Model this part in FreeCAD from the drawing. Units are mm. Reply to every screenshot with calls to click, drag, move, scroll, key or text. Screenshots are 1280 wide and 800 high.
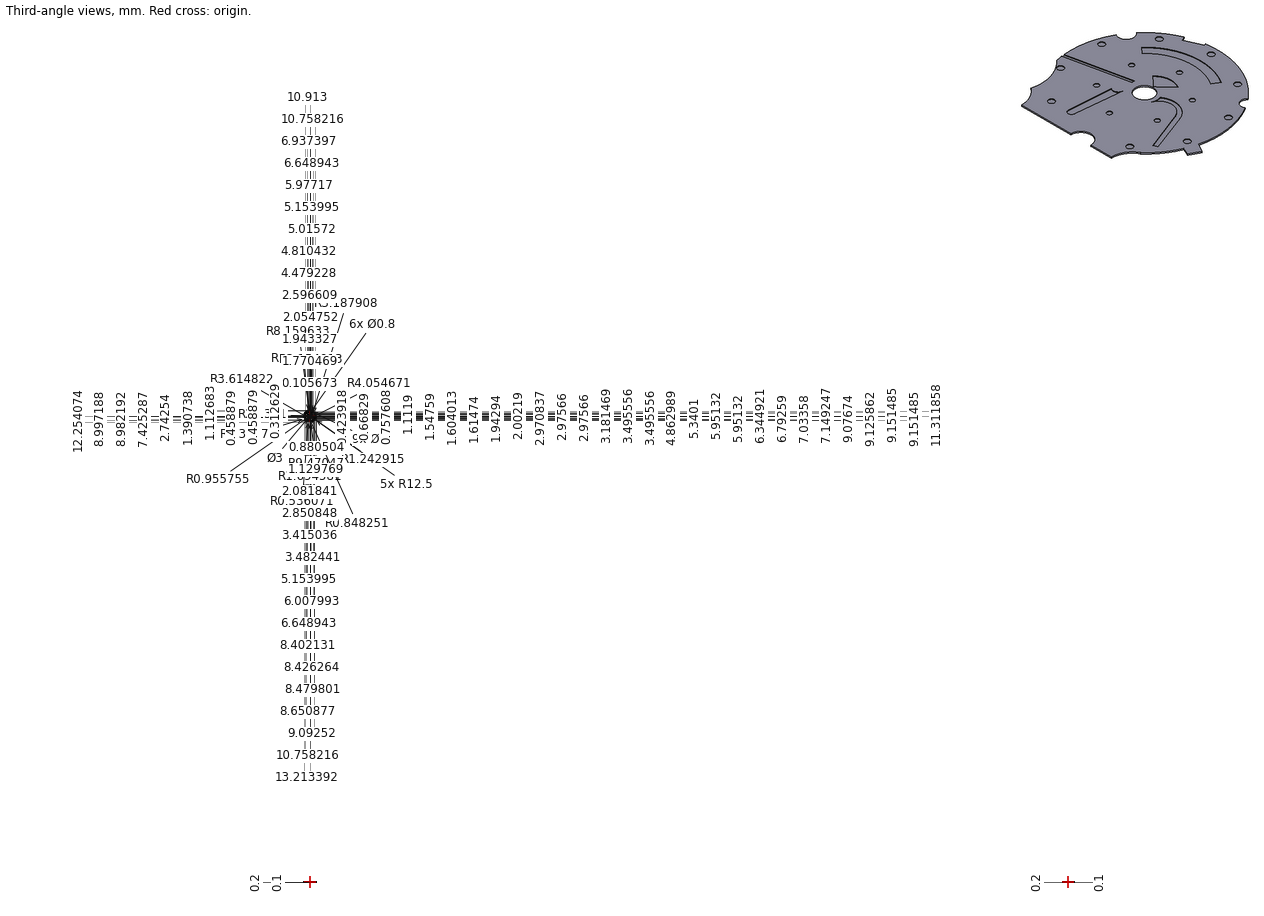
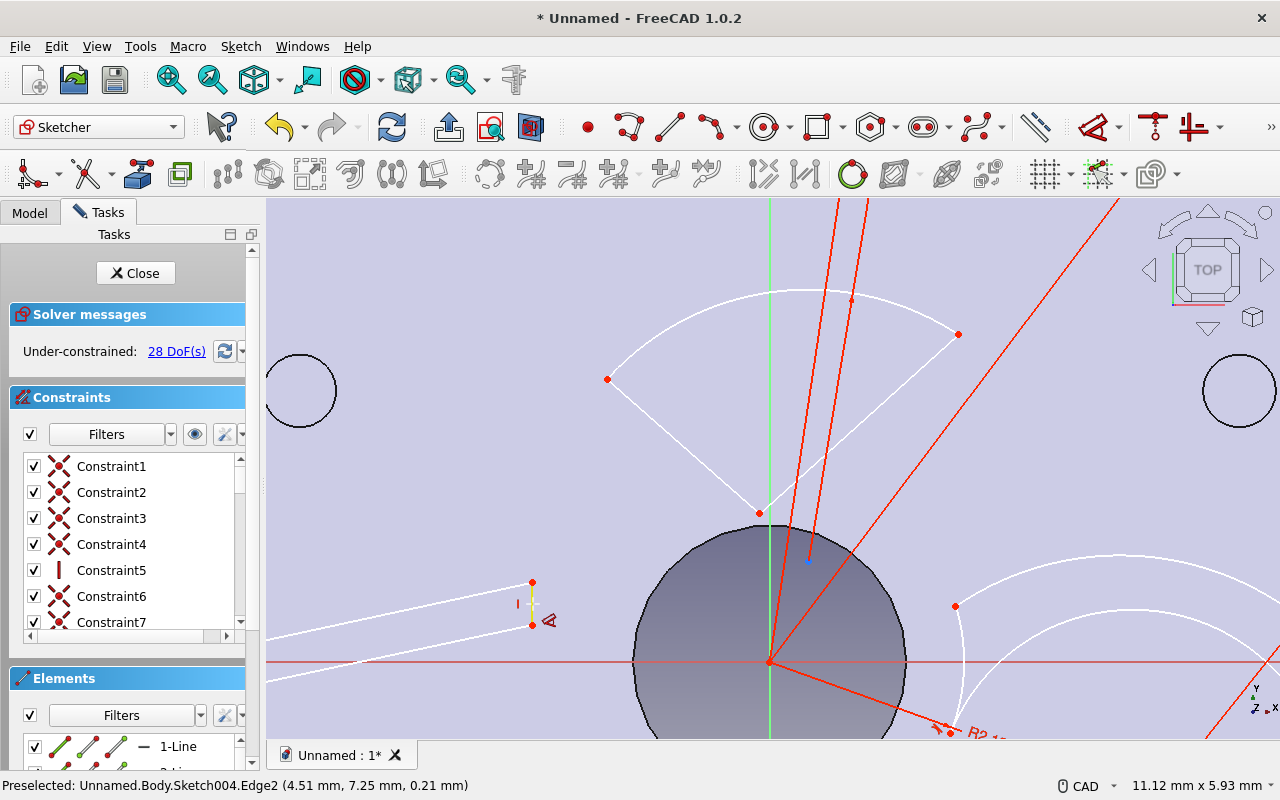
click(532, 604)
click(498, 604)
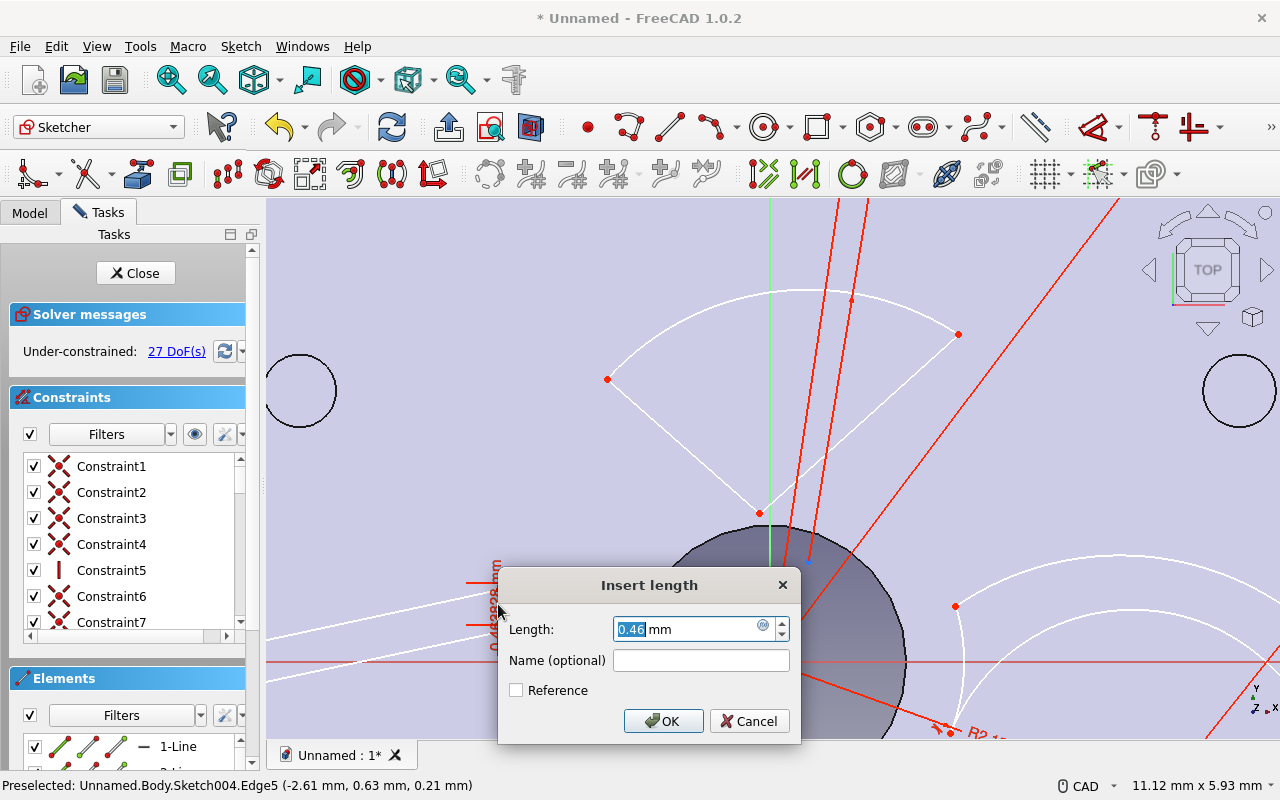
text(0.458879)
key(Return)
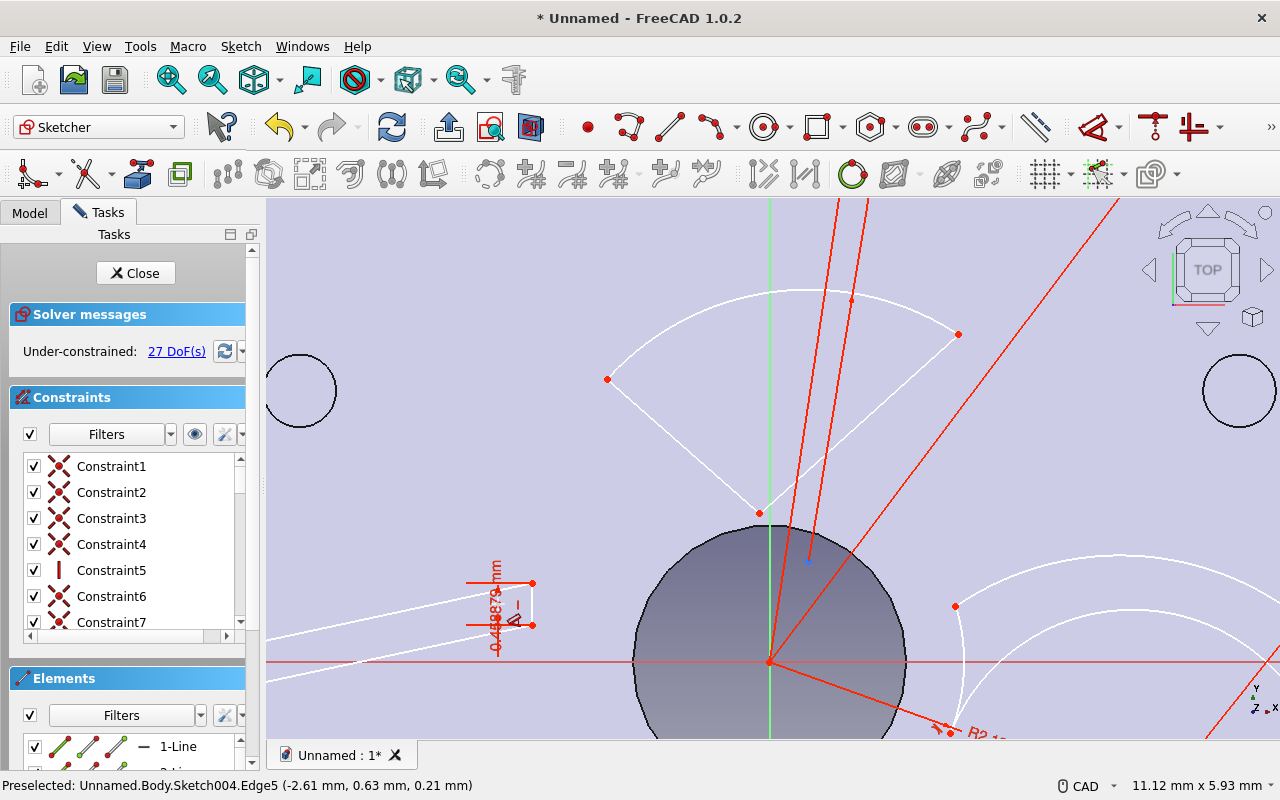
scroll(736, 417, down, 8)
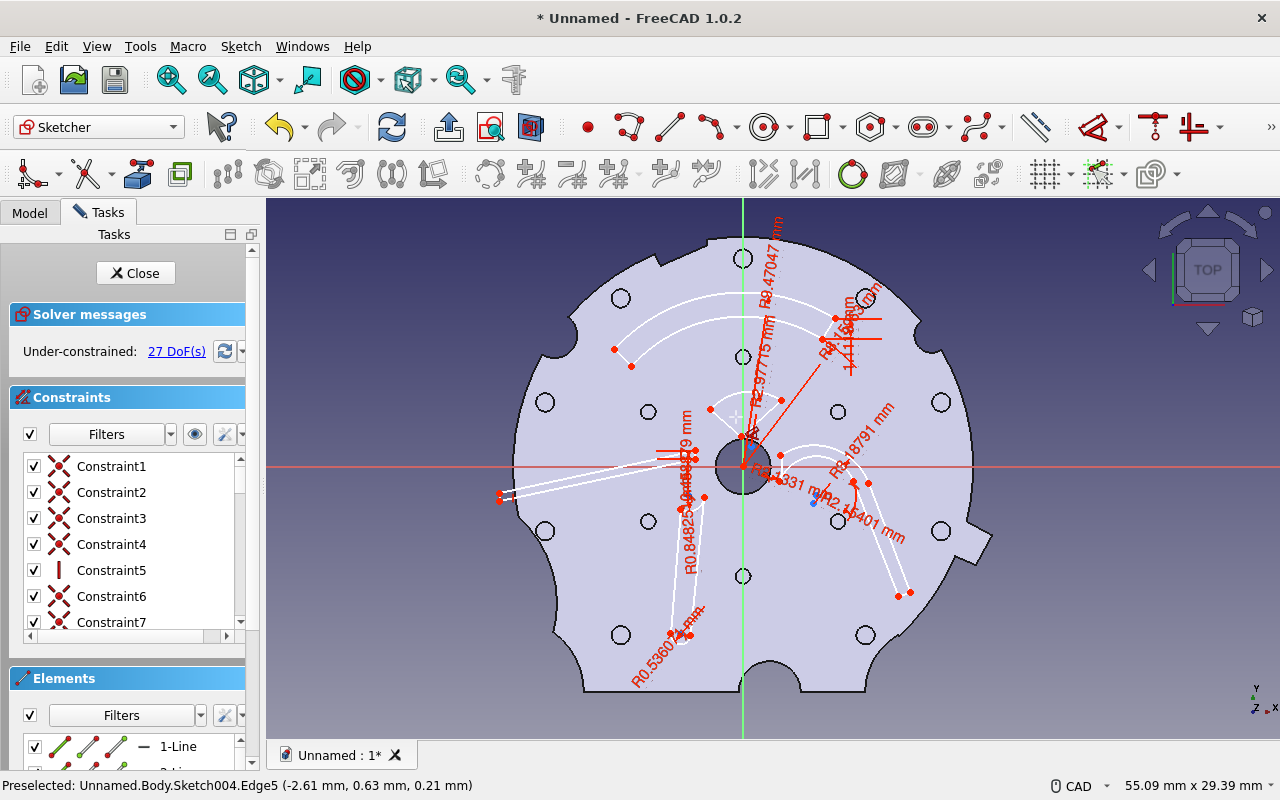
scroll(500, 495, up, 9)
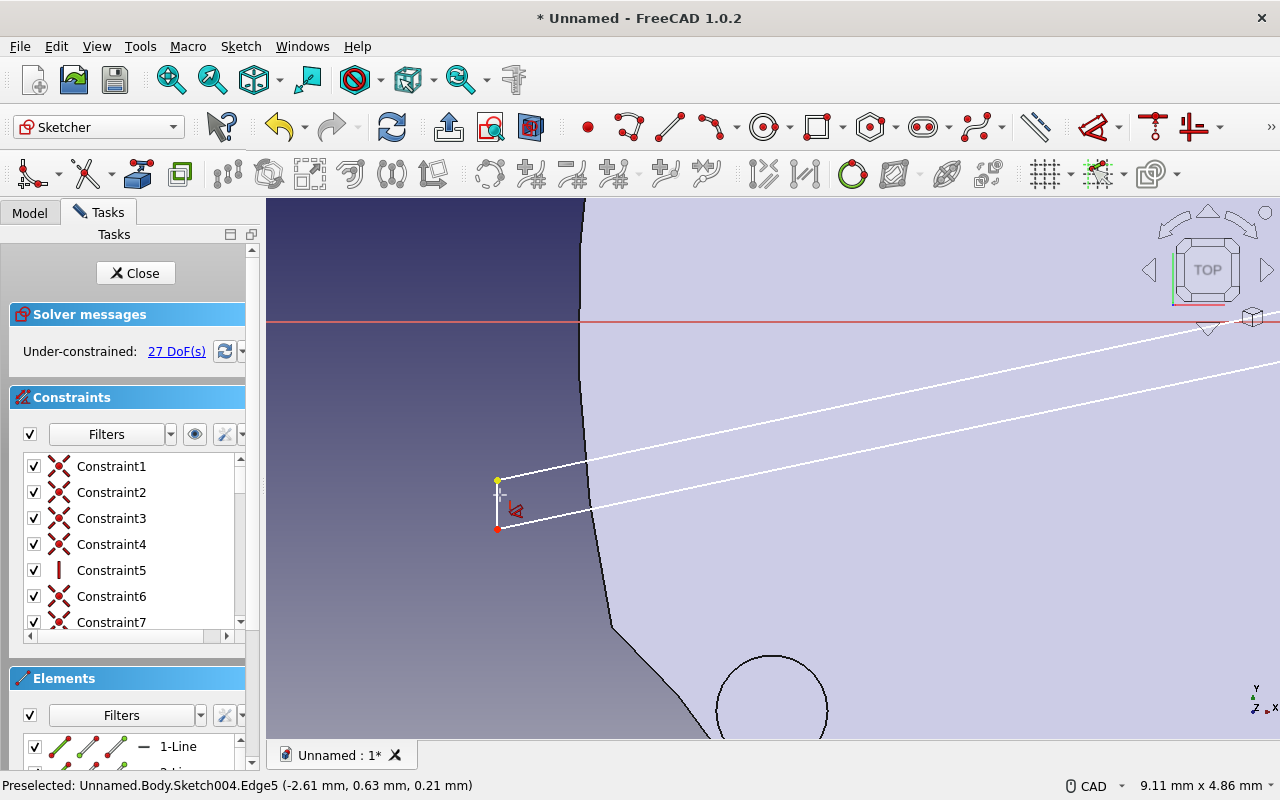
click(497, 495)
click(463, 505)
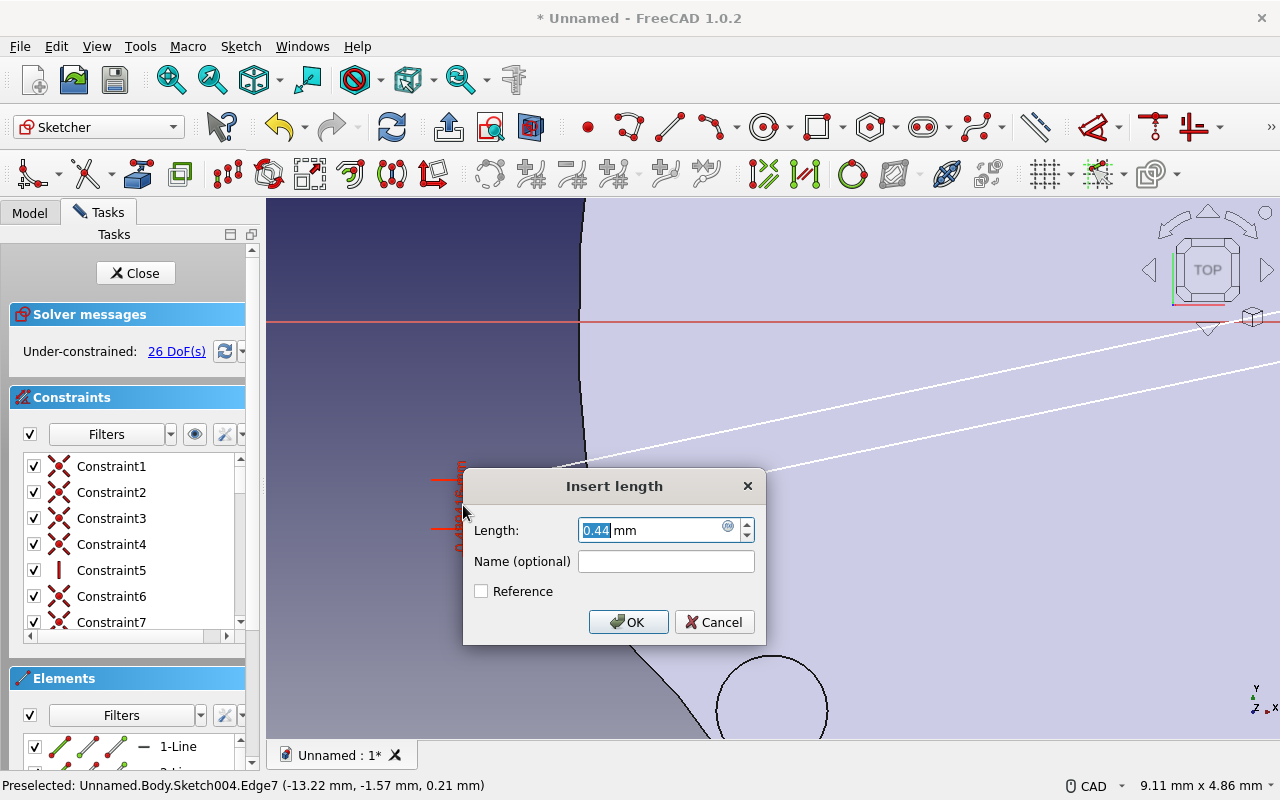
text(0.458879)
key(Return)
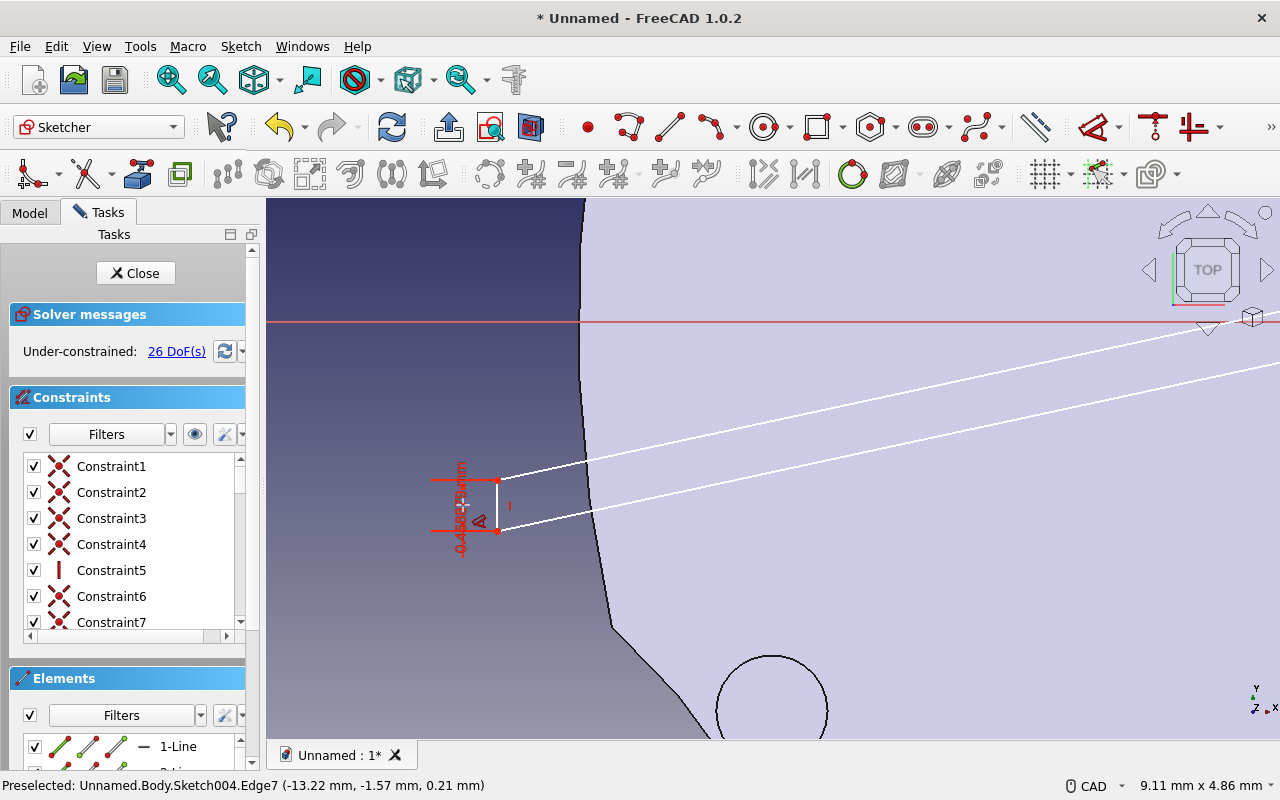
scroll(499, 496, down, 9)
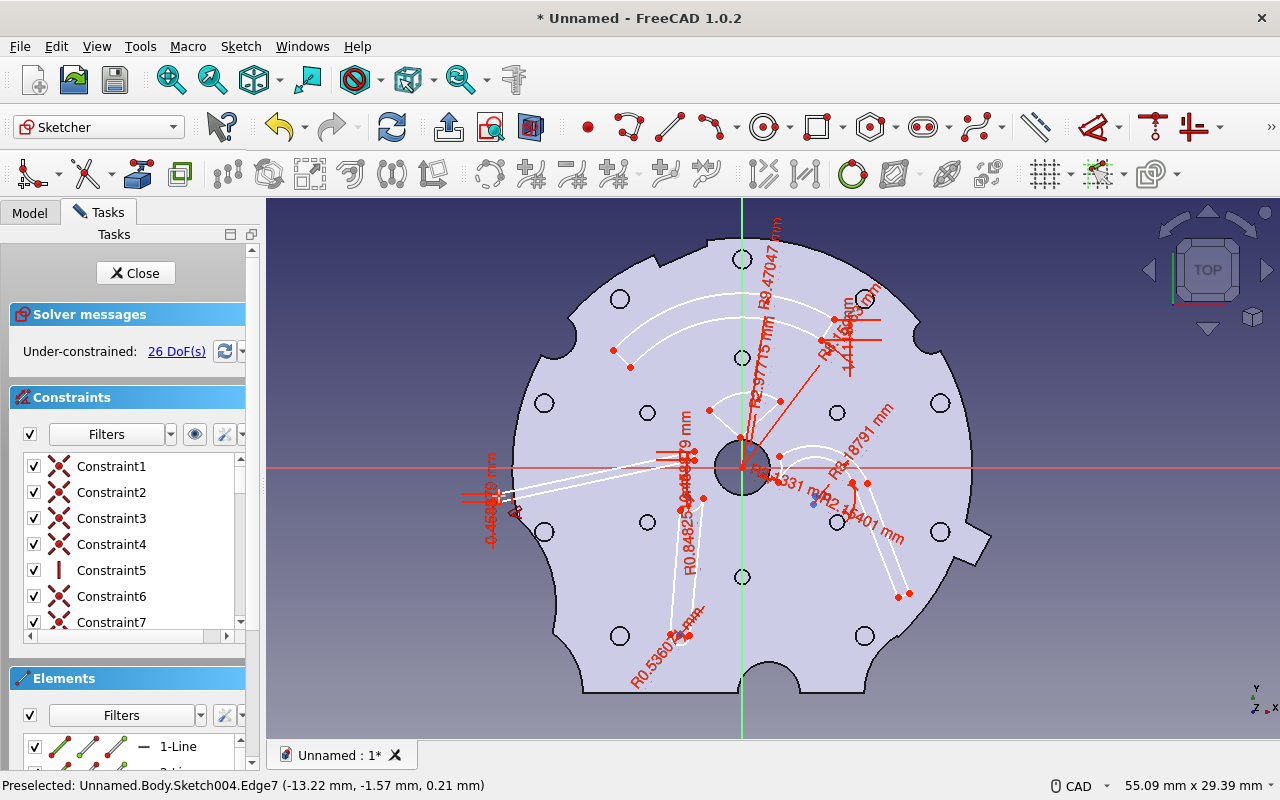
click(631, 367)
click(726, 333)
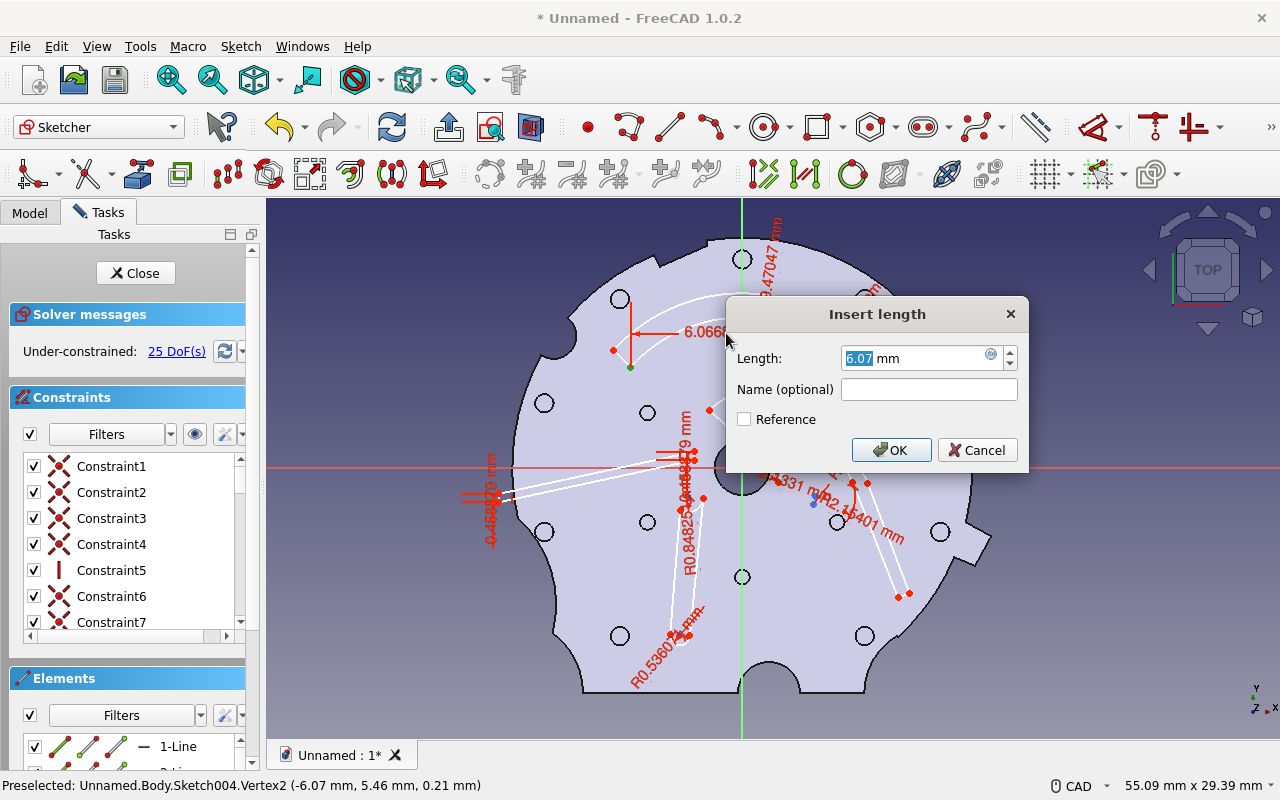
text(5.97717)
key(Return)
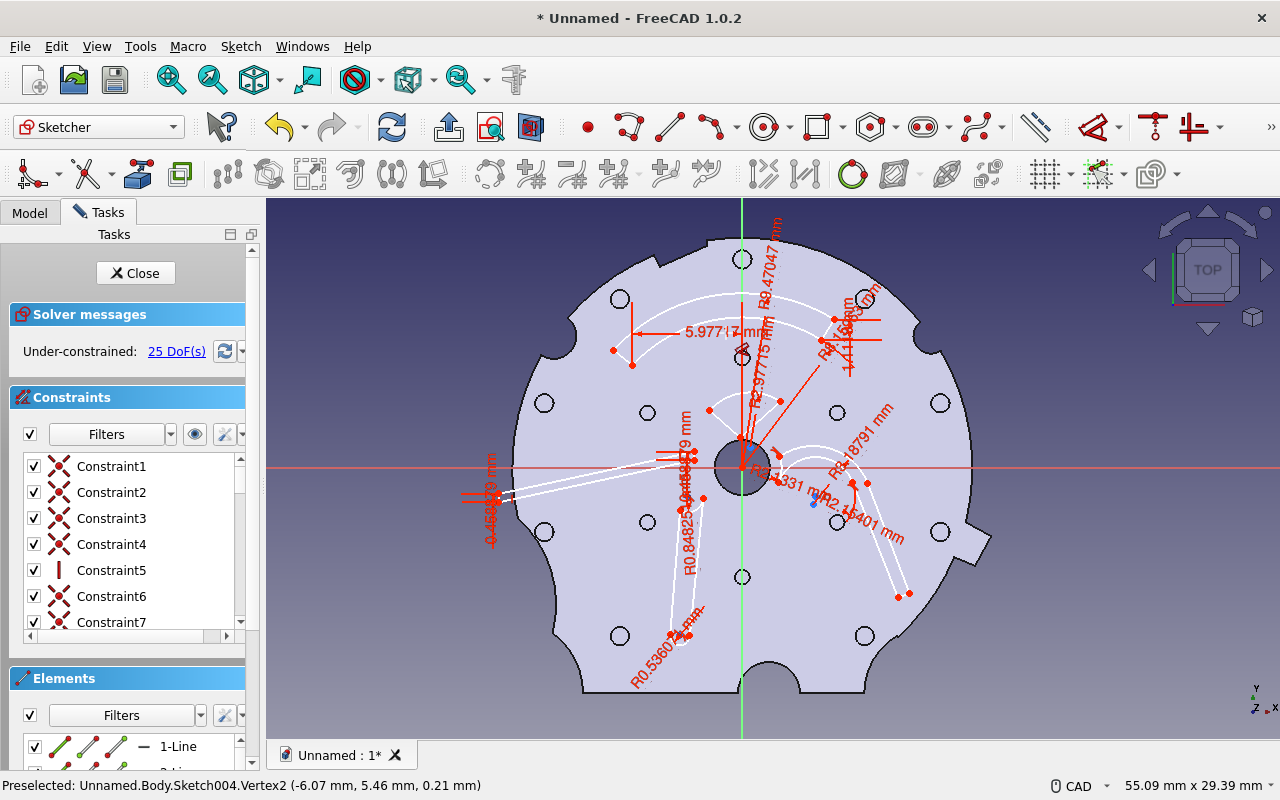
click(834, 320)
click(788, 286)